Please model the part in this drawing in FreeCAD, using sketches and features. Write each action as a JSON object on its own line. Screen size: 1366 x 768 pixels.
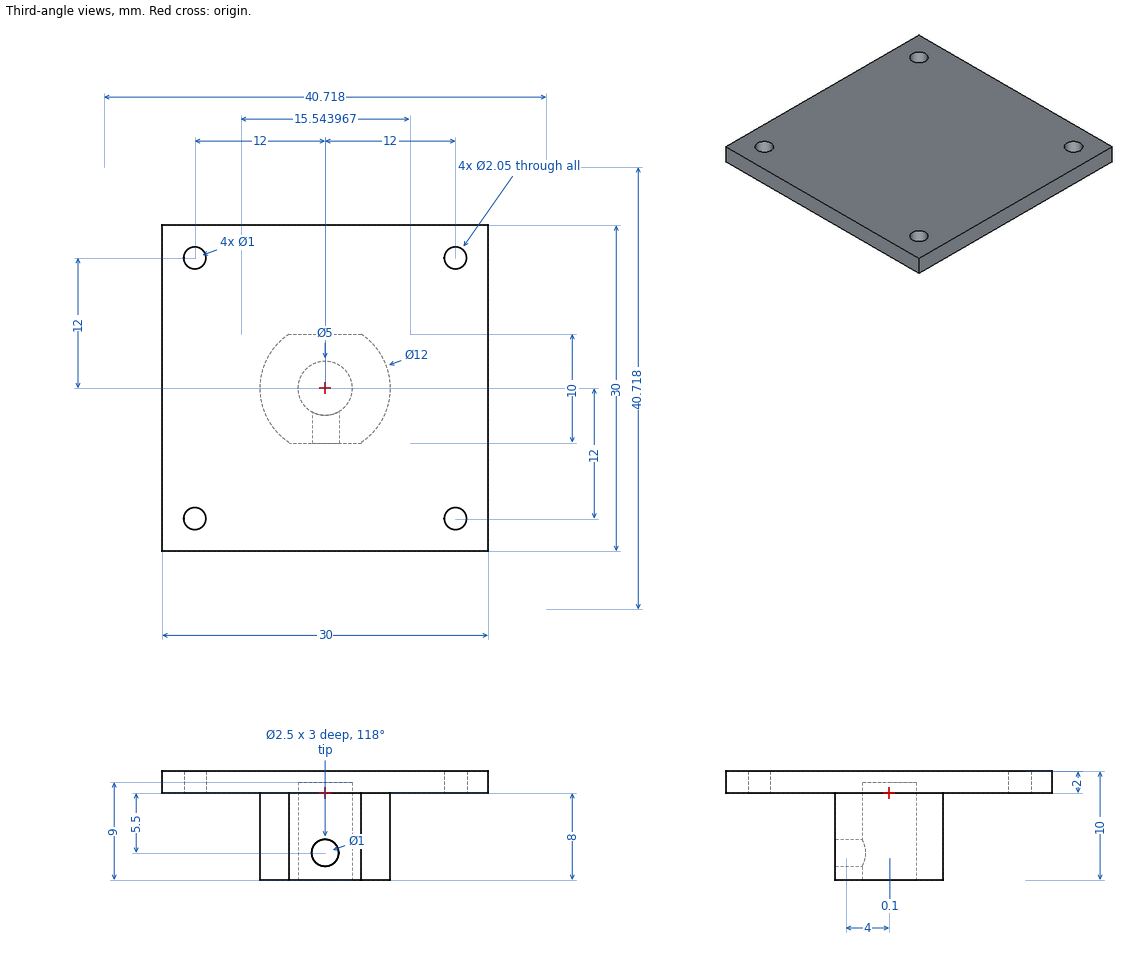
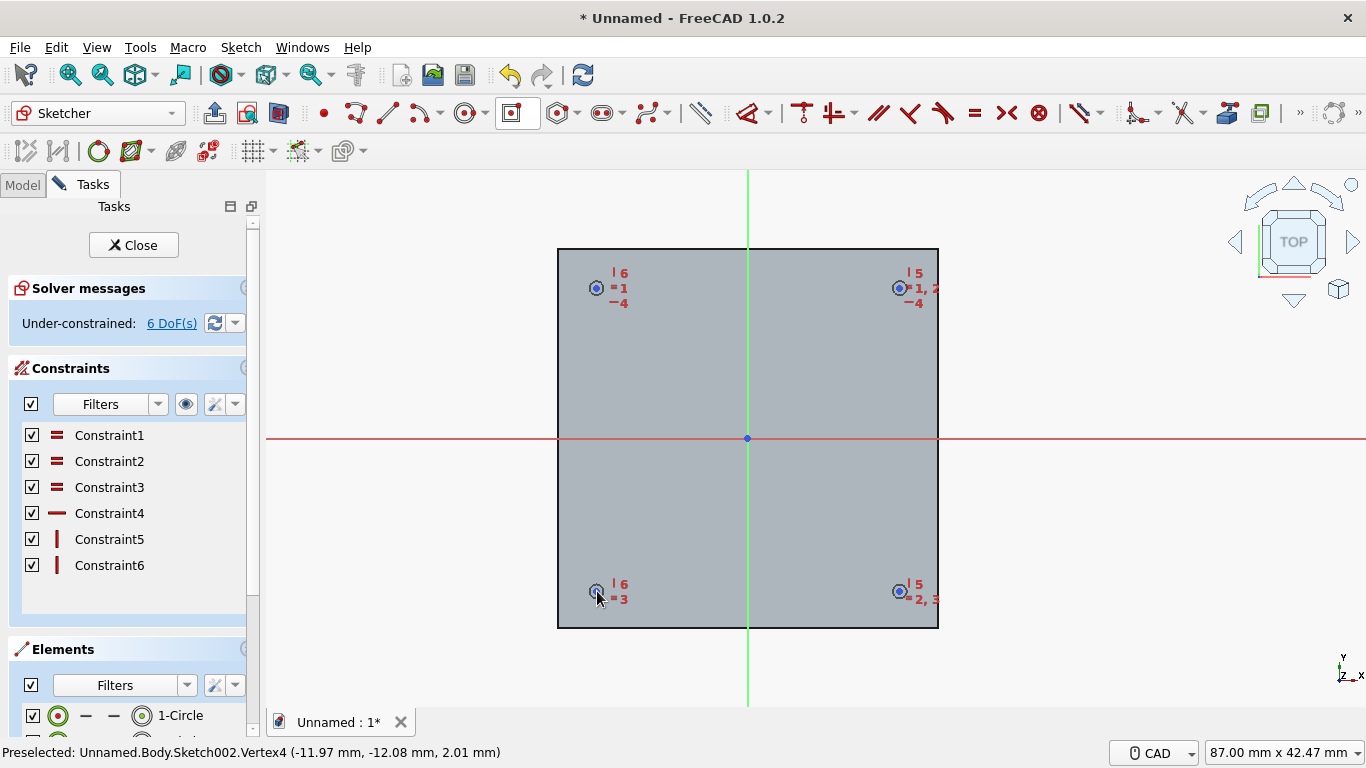
{"action": "left_click", "coordinate": [900, 591]}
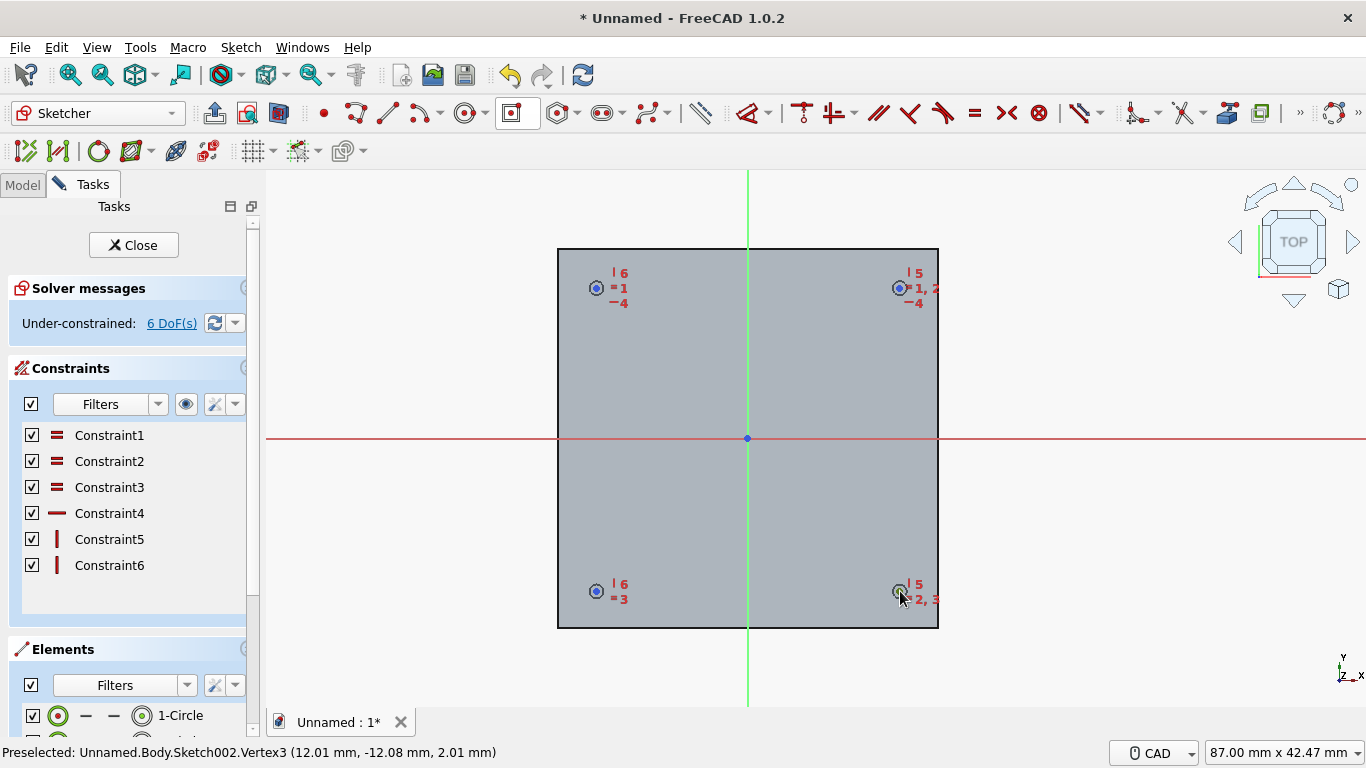
{"action": "left_click", "coordinate": [597, 591]}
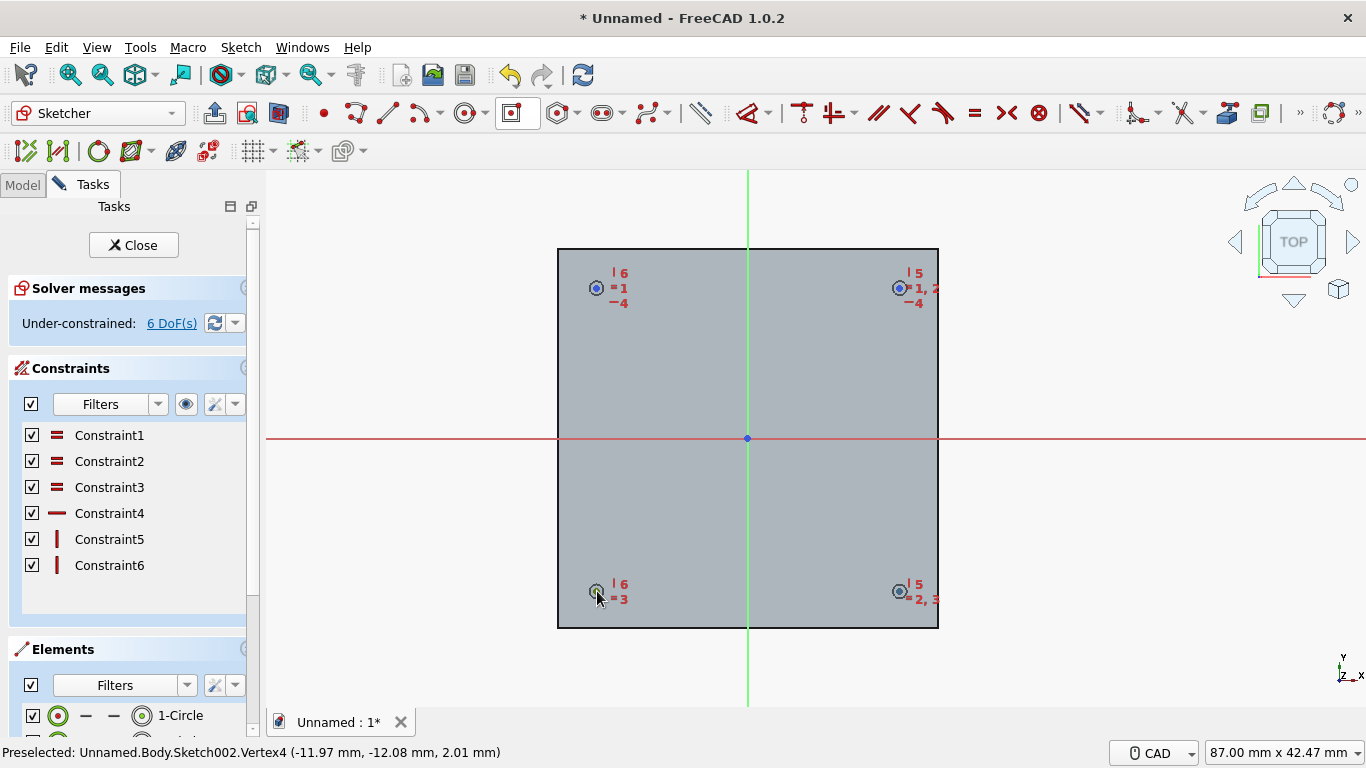
{"action": "left_click", "coordinate": [856, 114]}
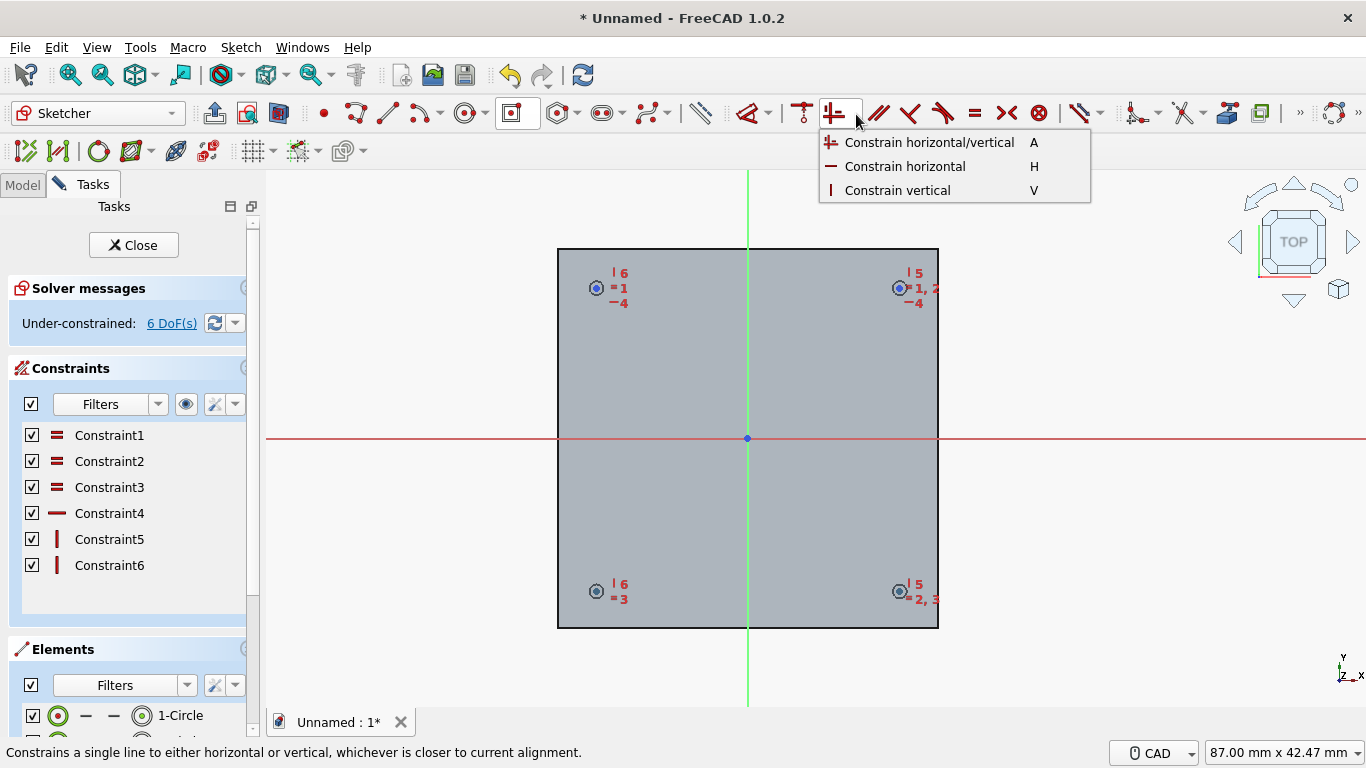
{"action": "left_click", "coordinate": [955, 166]}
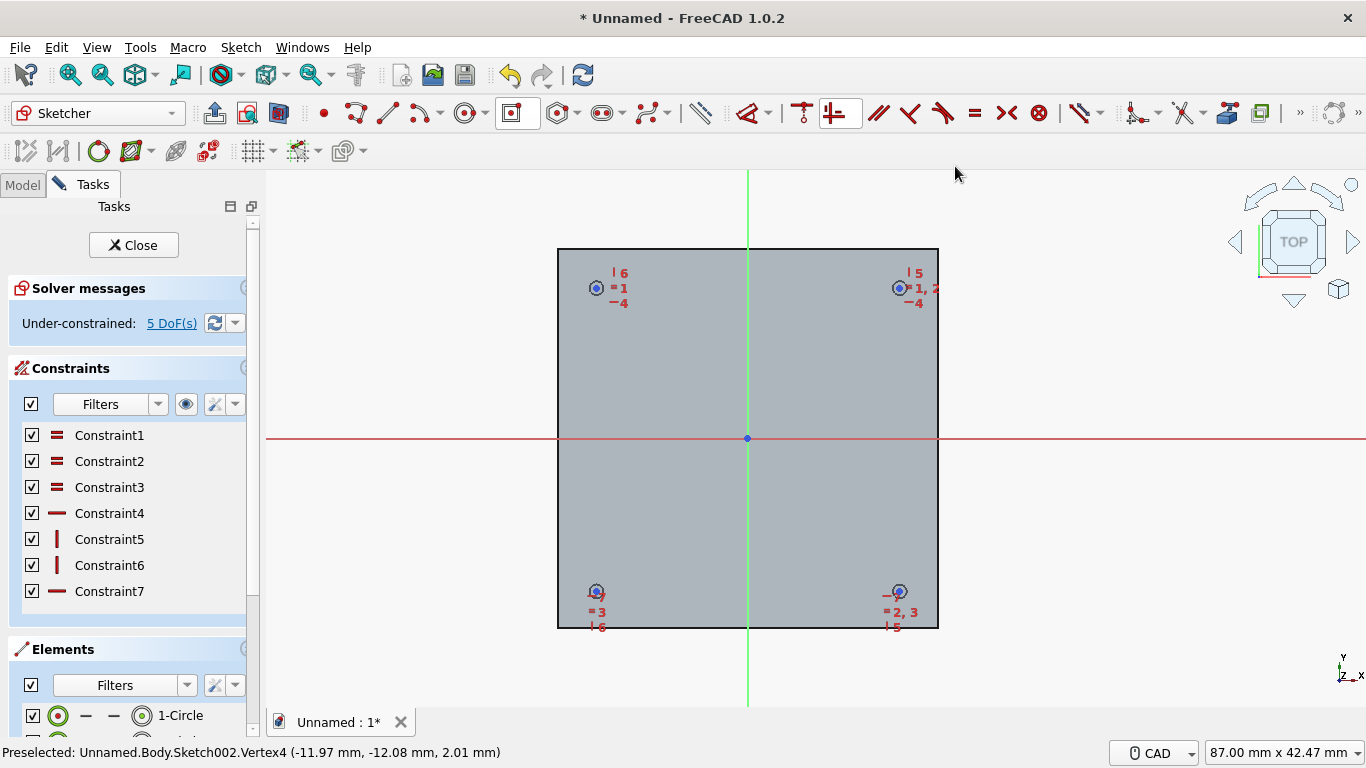
{"action": "key", "text": "d"}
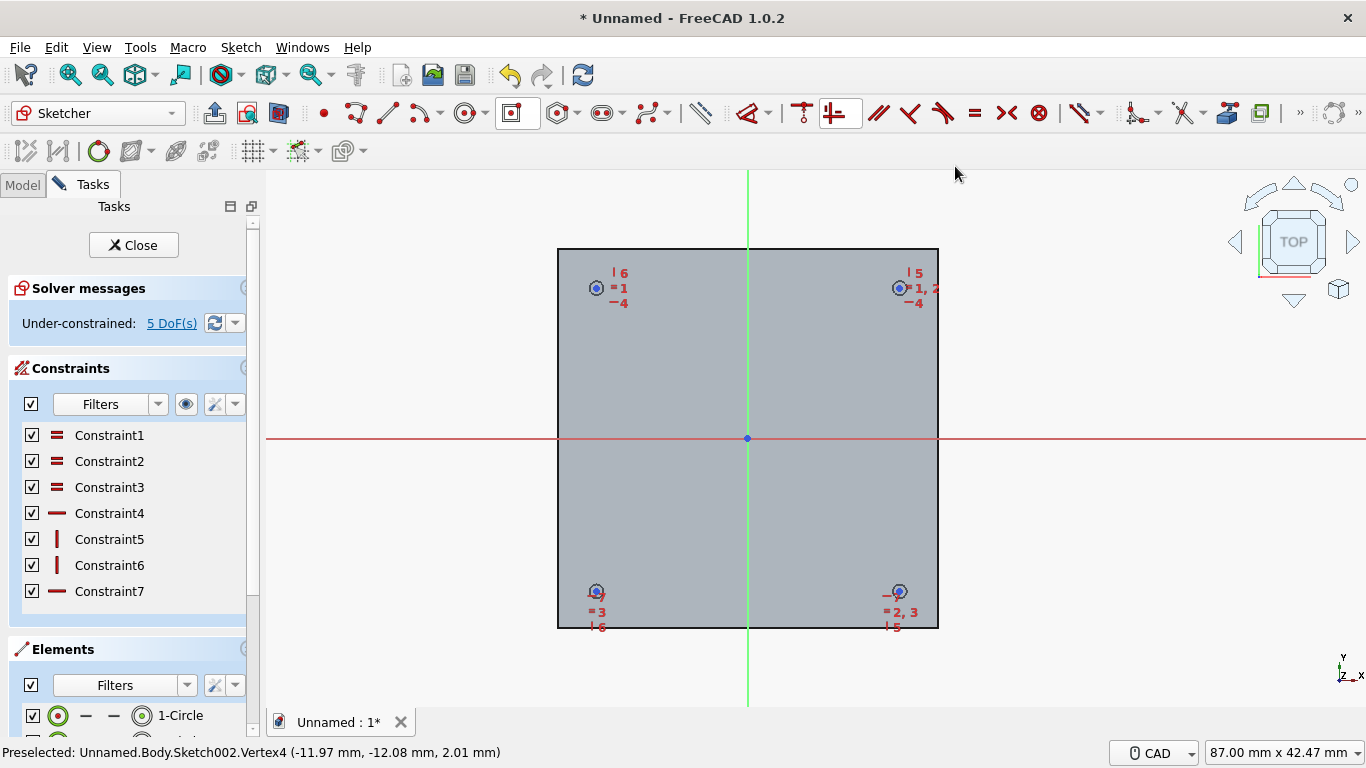
{"action": "scroll", "coordinate": [597, 281], "scroll_direction": "up", "scroll_amount": 6}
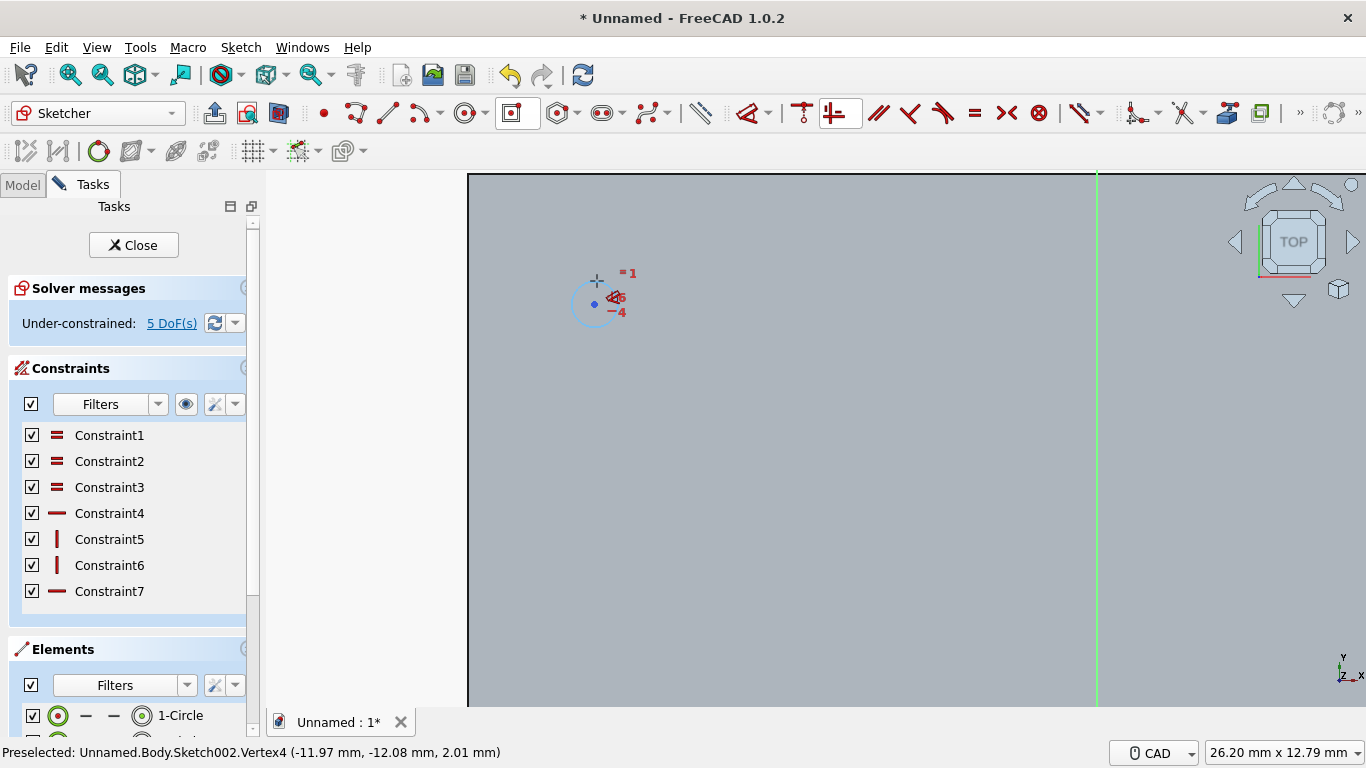
{"action": "left_click", "coordinate": [595, 281]}
{"action": "left_click", "coordinate": [595, 249]}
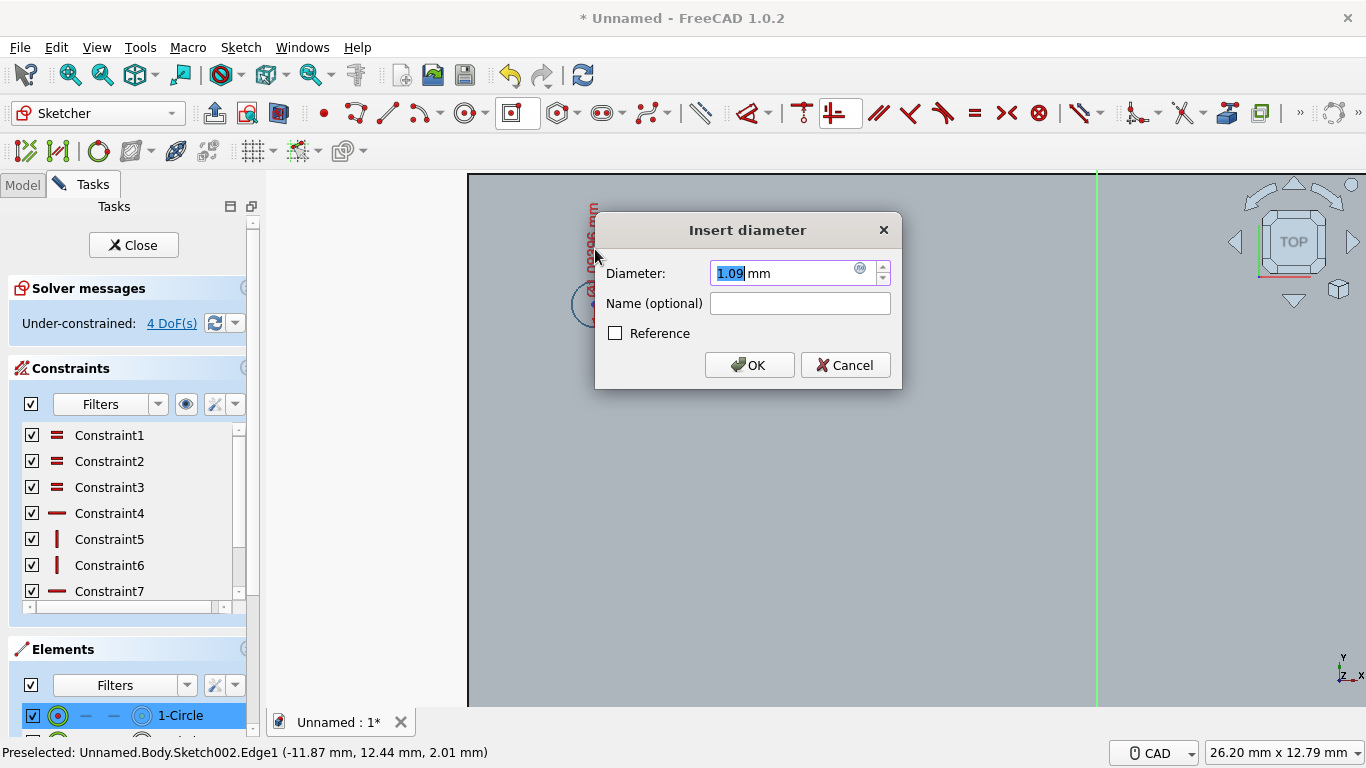
{"action": "type", "text": "1"}
{"action": "key", "text": "Return"}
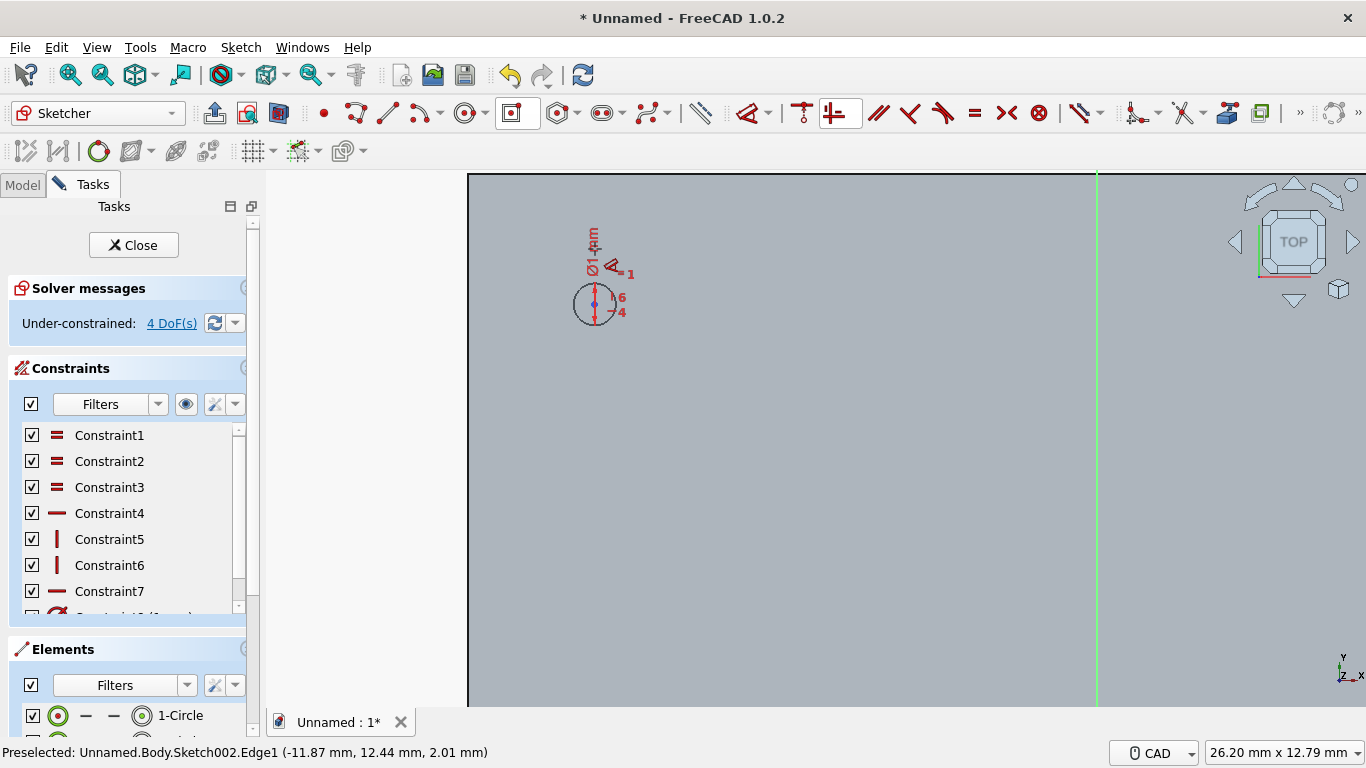
{"action": "left_click", "coordinate": [595, 304]}
{"action": "left_click", "coordinate": [846, 270]}